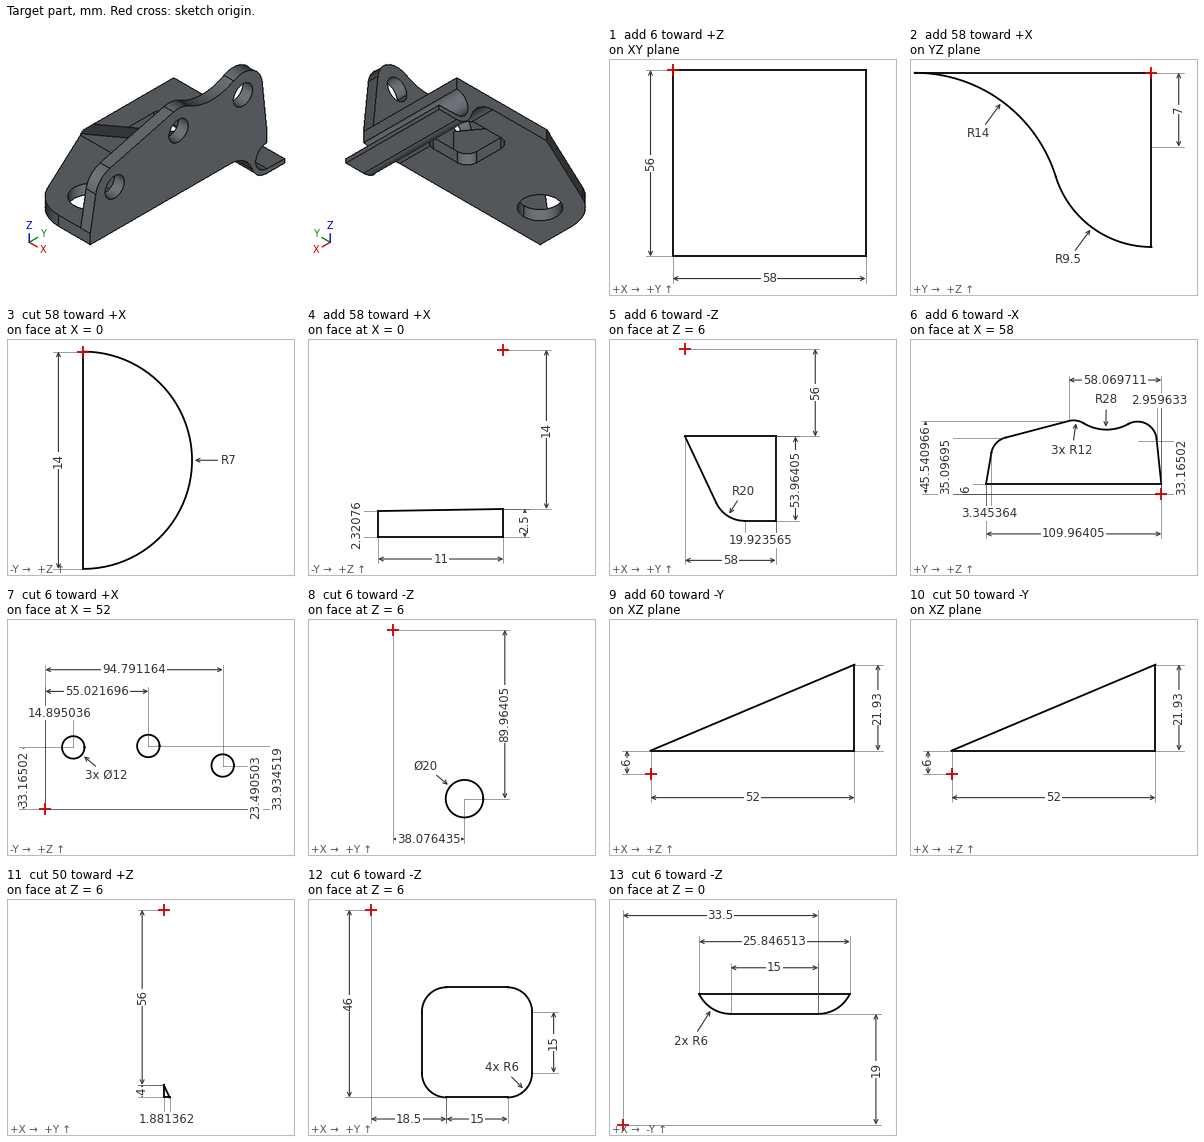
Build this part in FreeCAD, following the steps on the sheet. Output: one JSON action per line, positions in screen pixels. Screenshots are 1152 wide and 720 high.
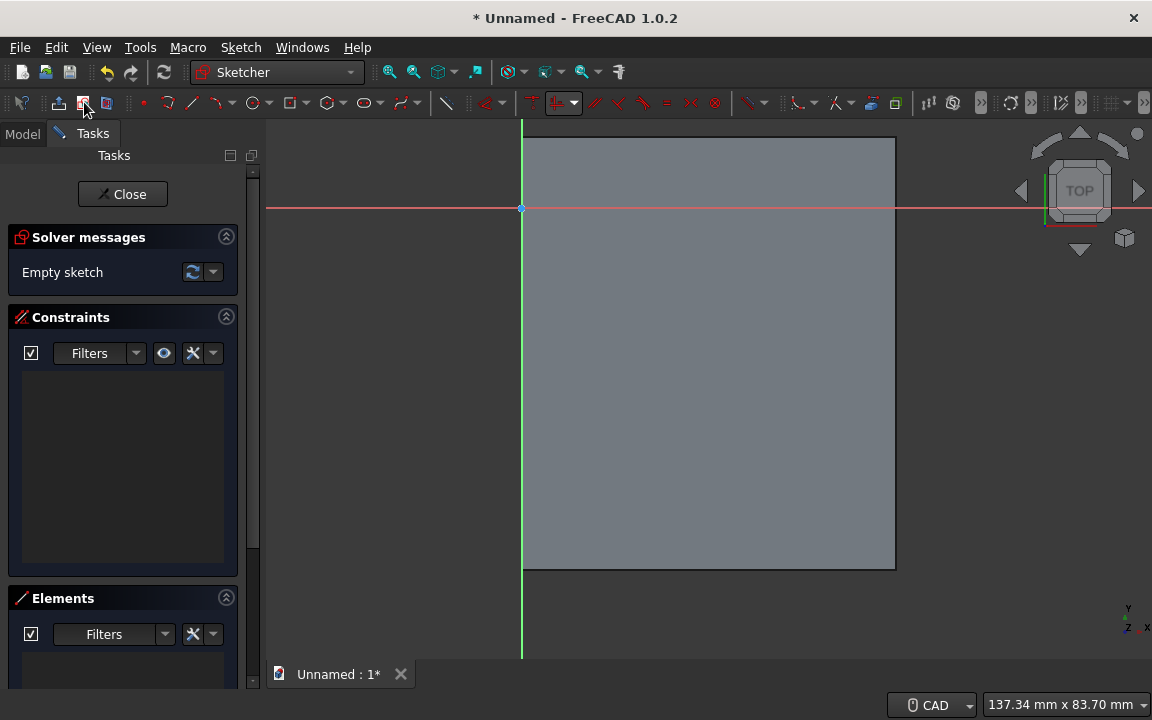
{"action": "scroll", "coordinate": [585, 247], "scroll_direction": "down", "scroll_amount": 4}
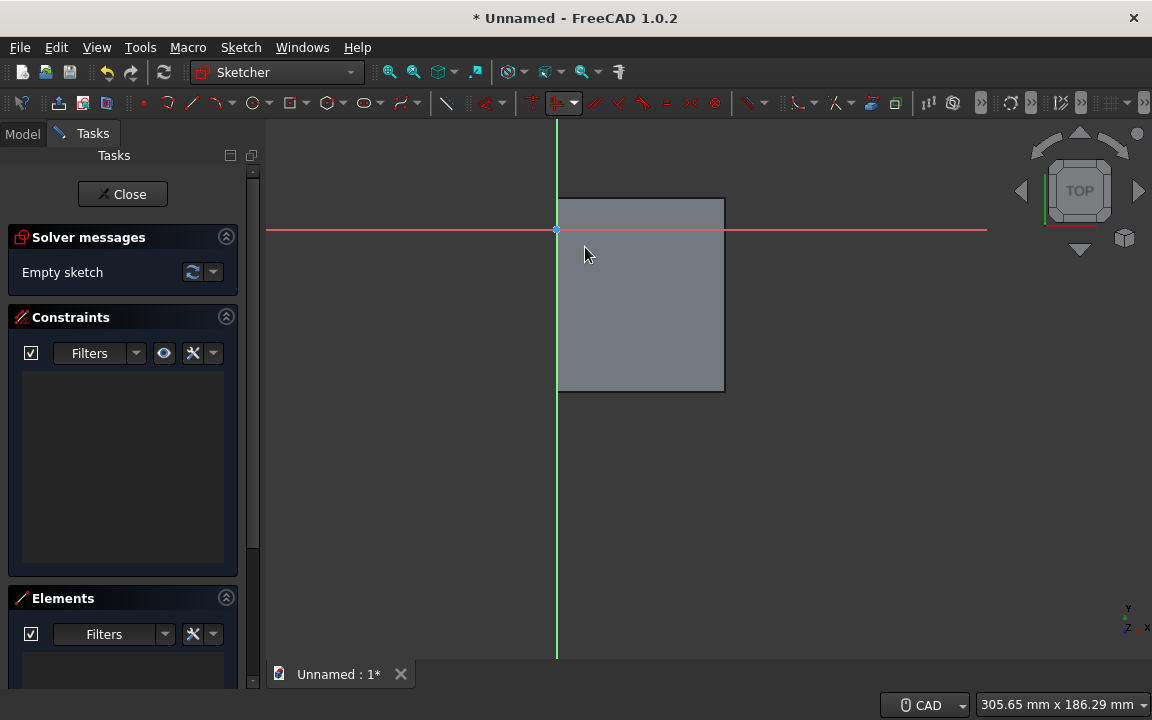
{"action": "left_click", "coordinate": [168, 104]}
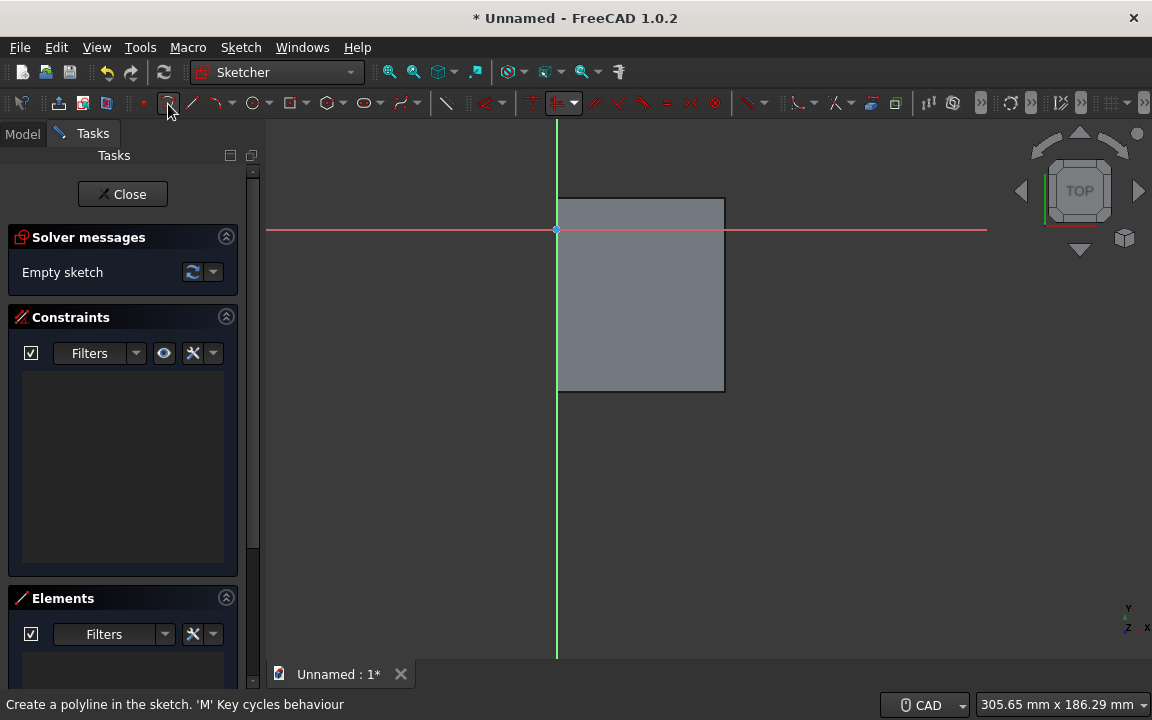
{"action": "left_click", "coordinate": [667, 549]}
{"action": "left_click", "coordinate": [725, 549]}
{"action": "left_click", "coordinate": [725, 392]}
{"action": "left_click", "coordinate": [557, 392]}
{"action": "left_click", "coordinate": [615, 515]}
{"action": "right_click", "coordinate": [615, 515]}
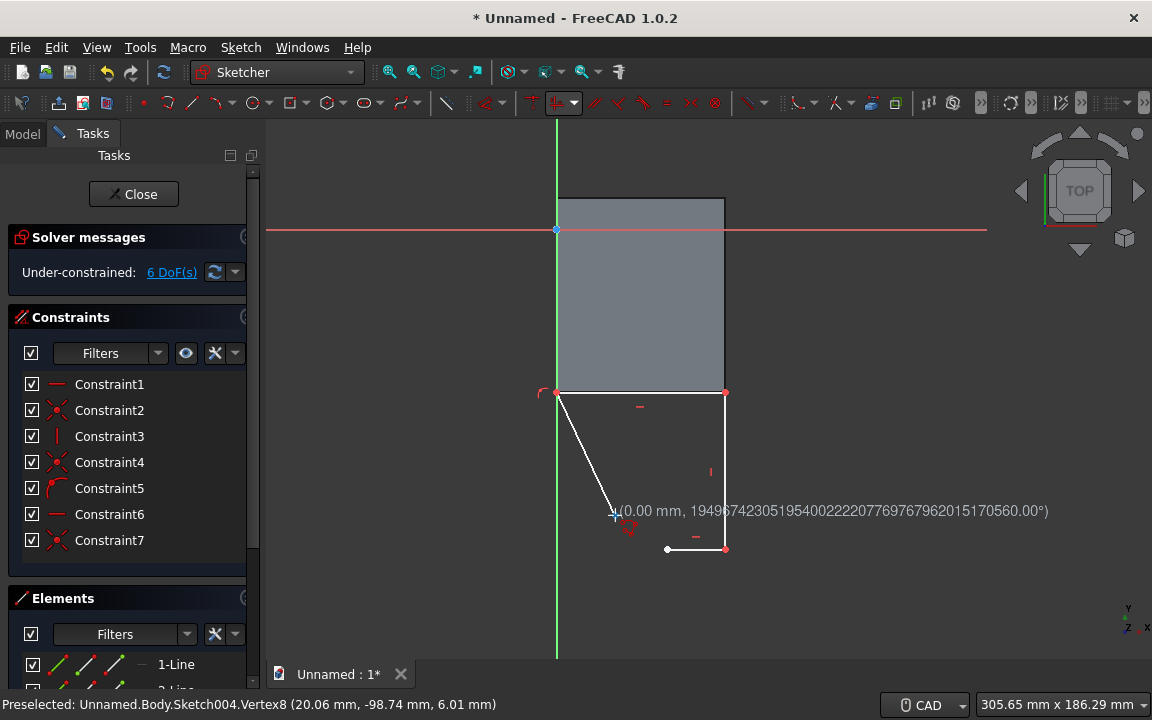
{"action": "key", "text": "g 3 a"}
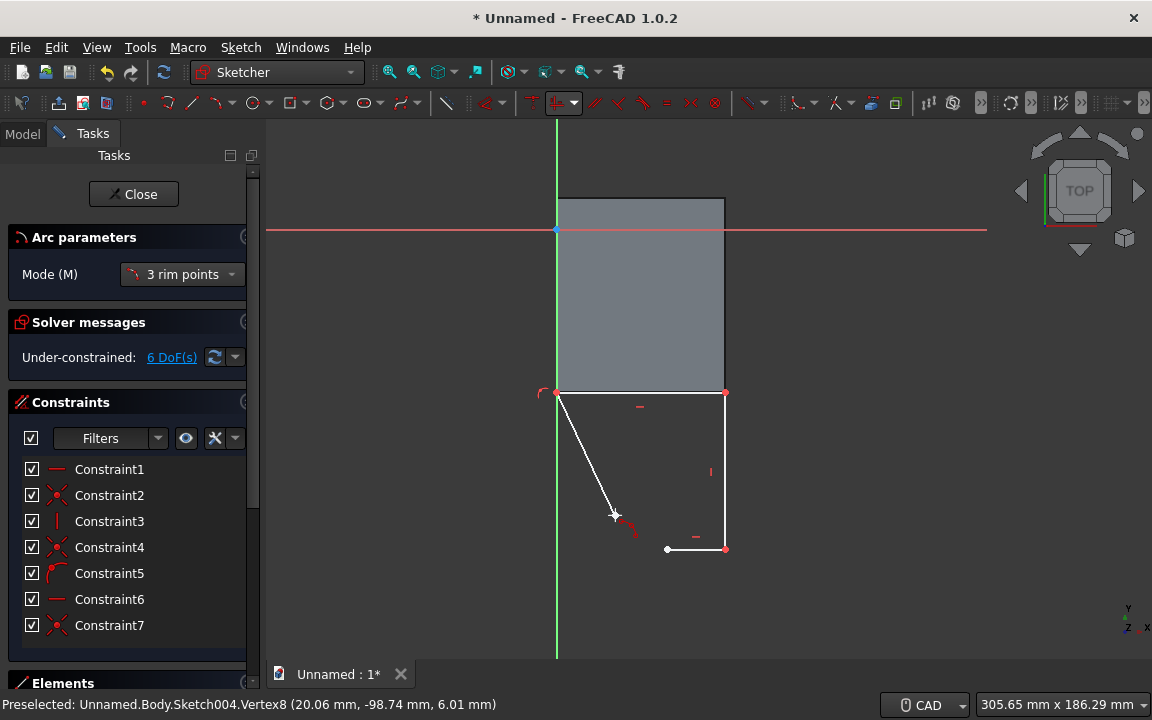
{"action": "left_click", "coordinate": [615, 516]}
{"action": "left_click", "coordinate": [667, 550]}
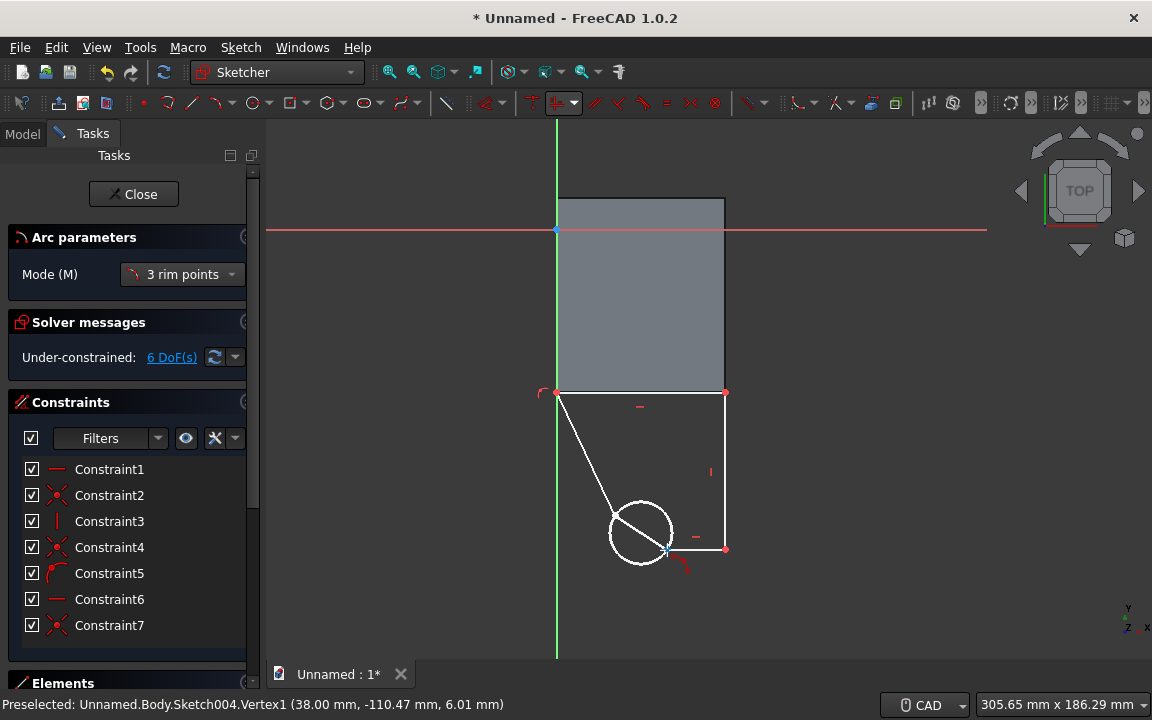
{"action": "scroll", "coordinate": [636, 540], "scroll_direction": "up", "scroll_amount": 3}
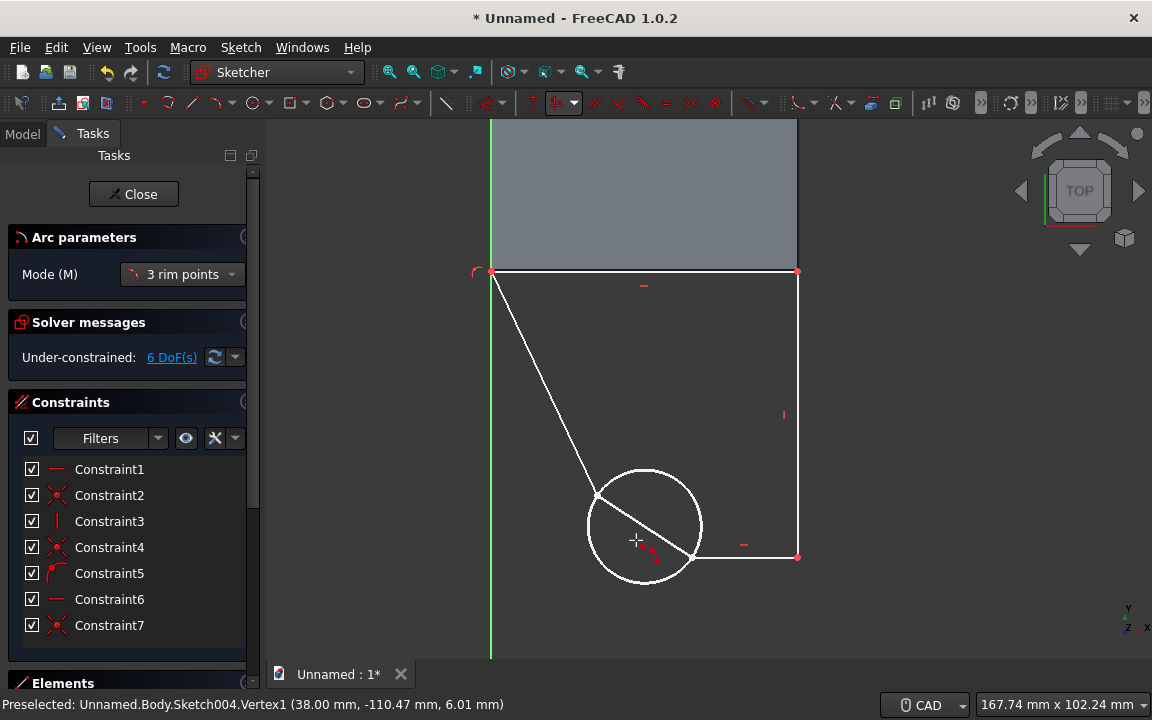
{"action": "left_click", "coordinate": [636, 538]}
{"action": "key", "text": "Escape"}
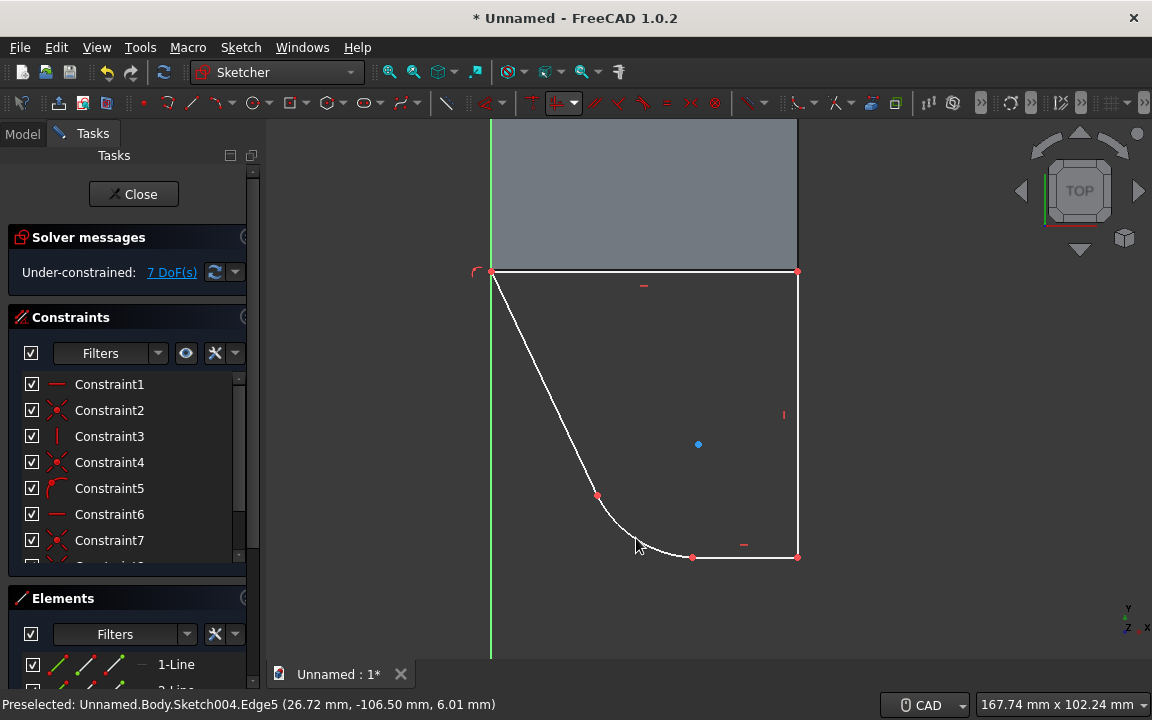
{"action": "left_click", "coordinate": [724, 558]}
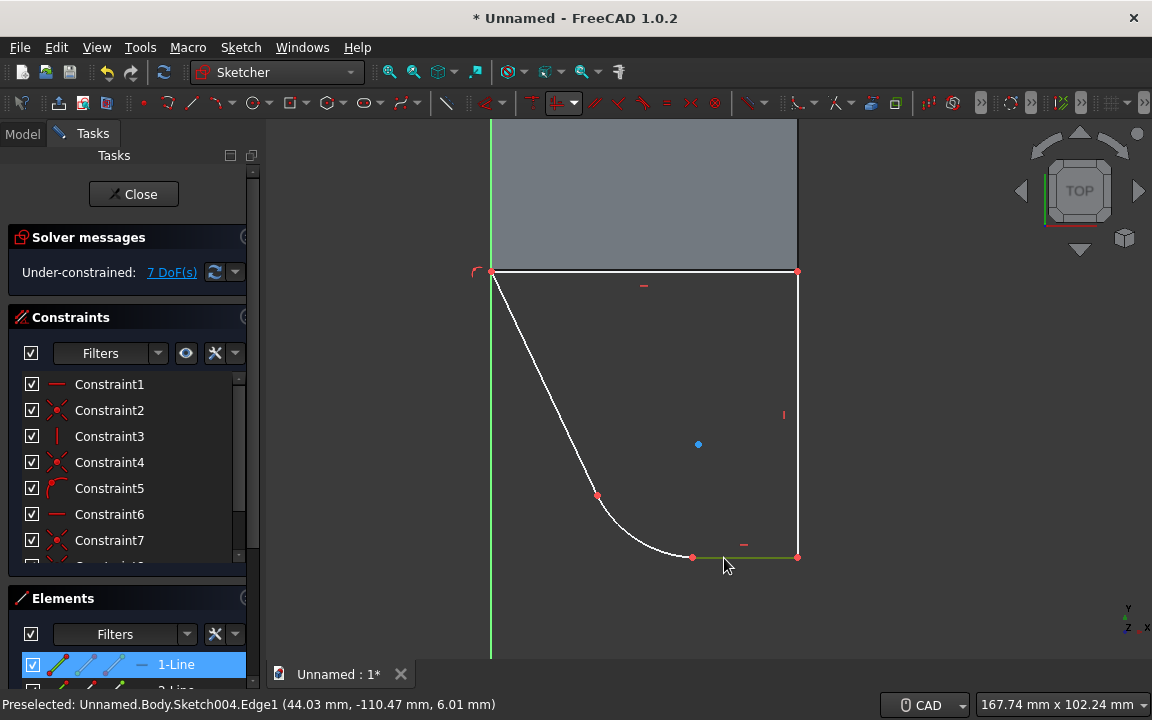
{"action": "left_click", "coordinate": [618, 524]}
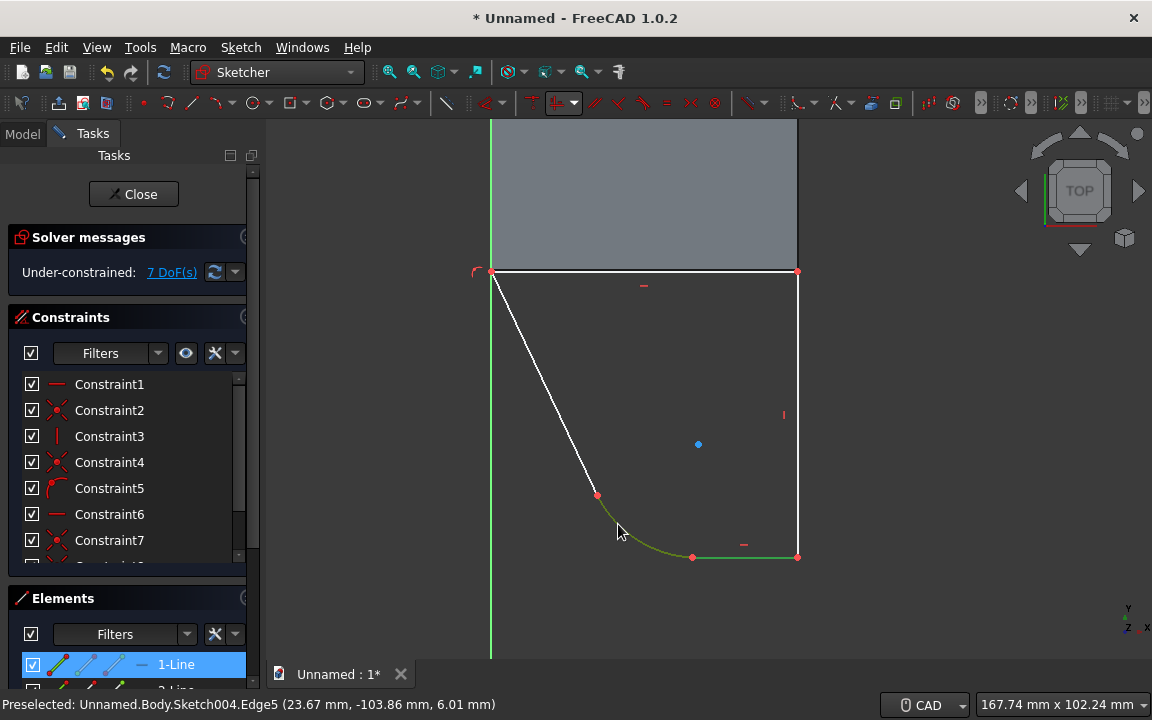
{"action": "left_click", "coordinate": [644, 104]}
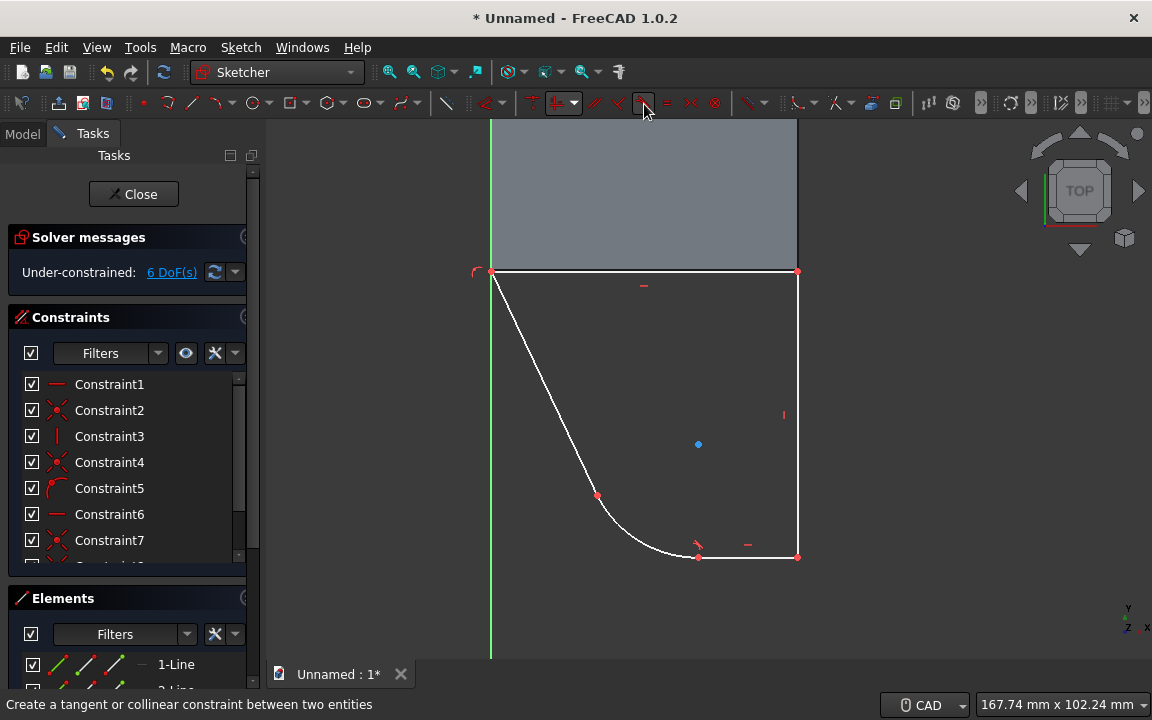
{"action": "left_click", "coordinate": [523, 339]}